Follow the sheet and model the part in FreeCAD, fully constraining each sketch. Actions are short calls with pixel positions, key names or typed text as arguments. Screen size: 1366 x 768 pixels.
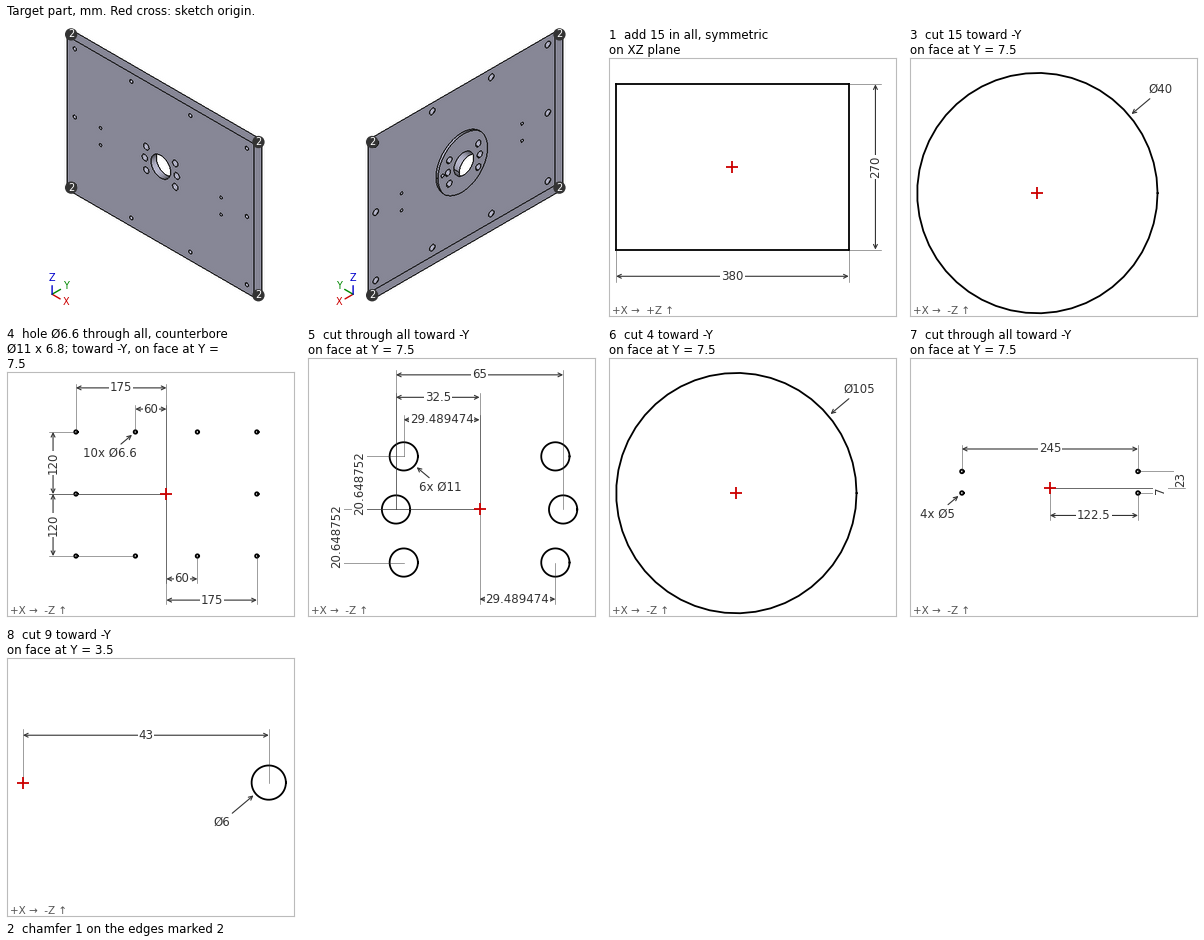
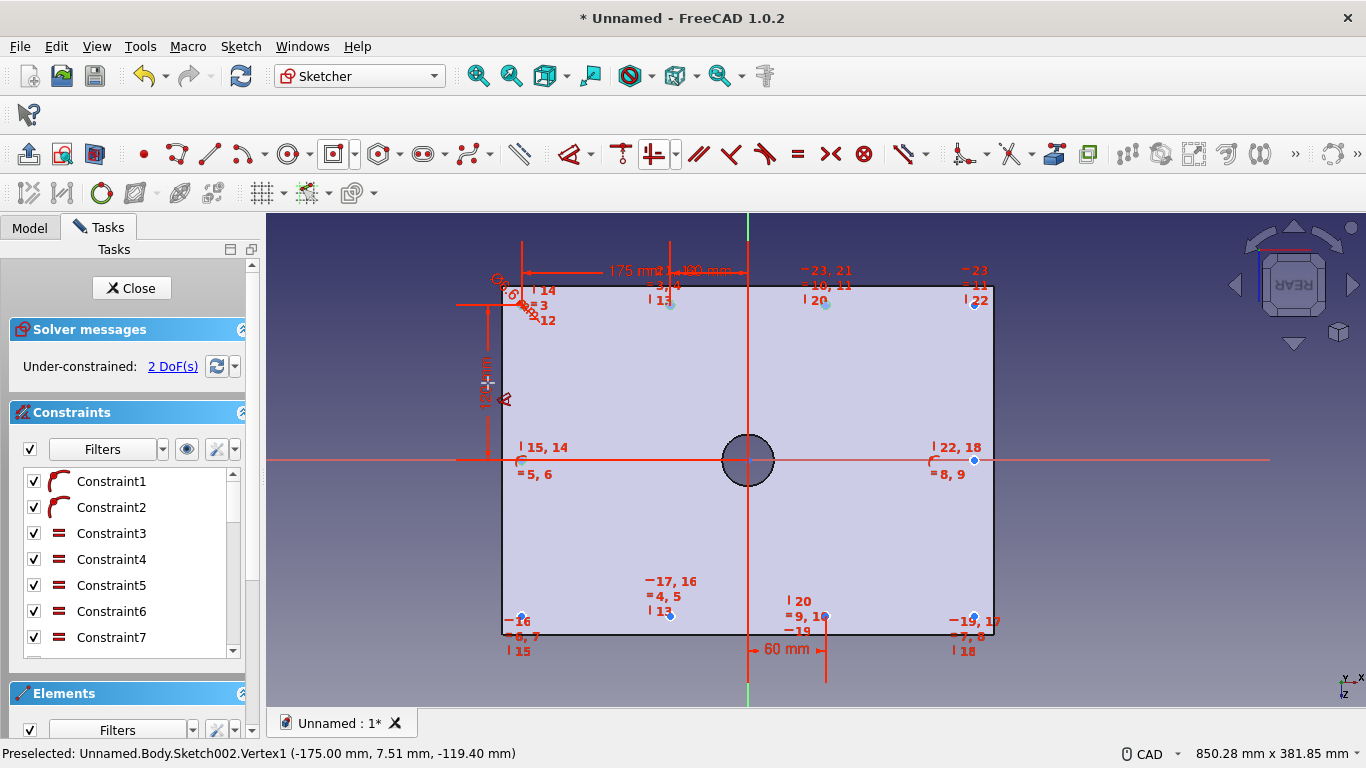
click(670, 616)
click(636, 538)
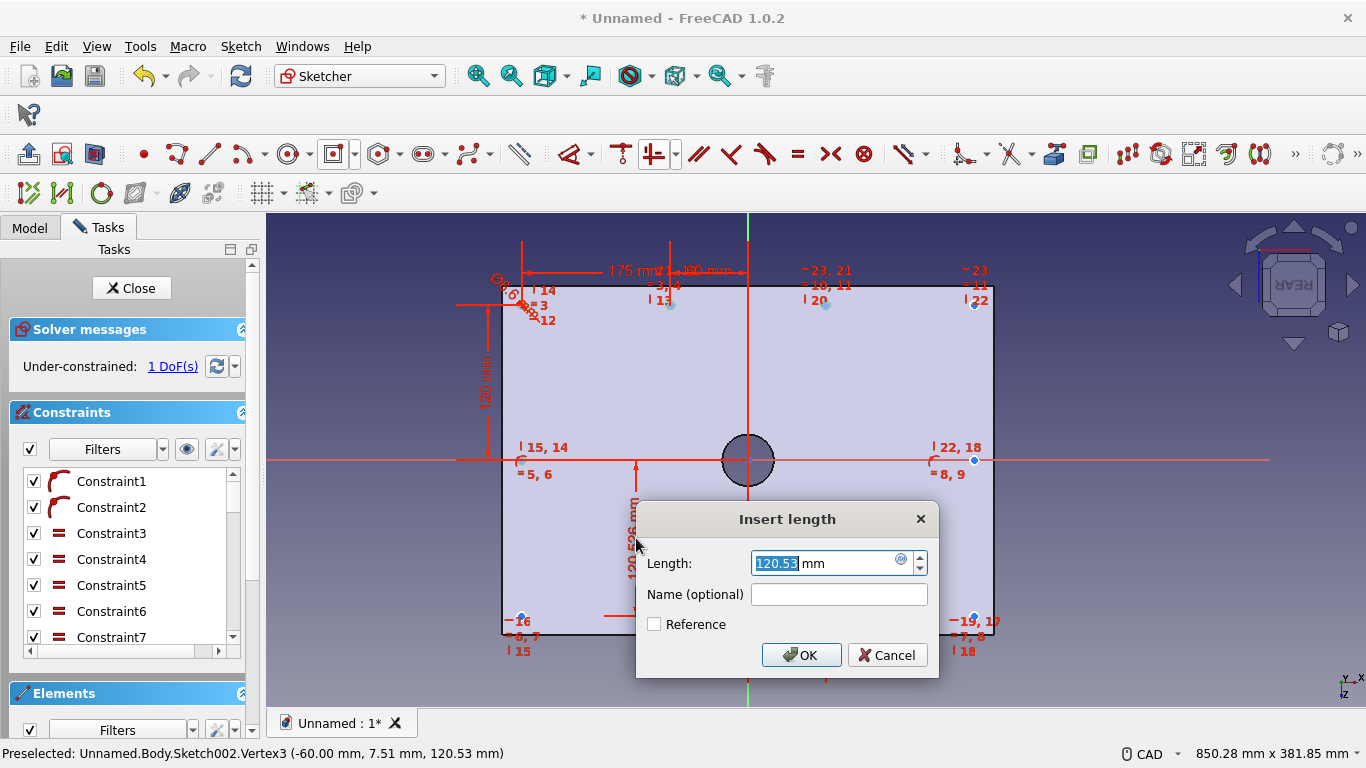
text(120)
key(Return)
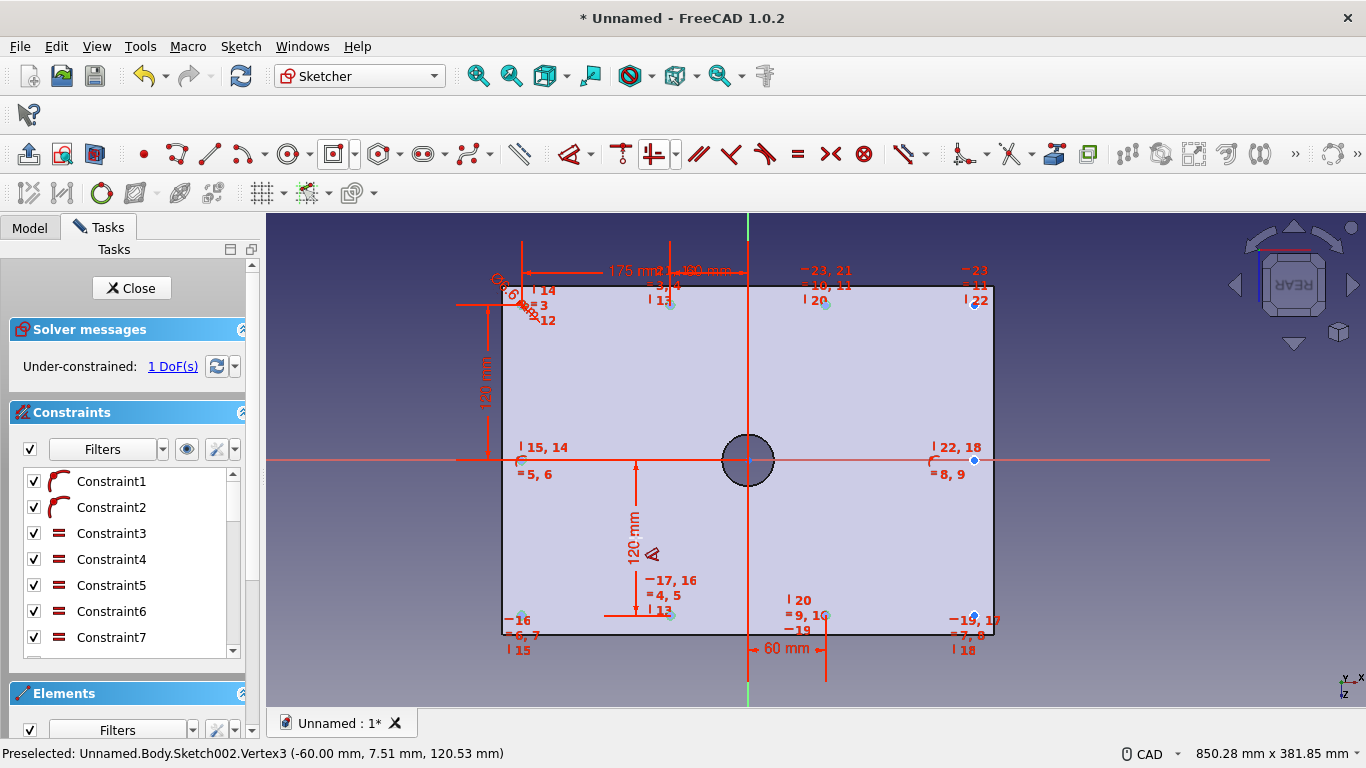
click(974, 616)
click(861, 650)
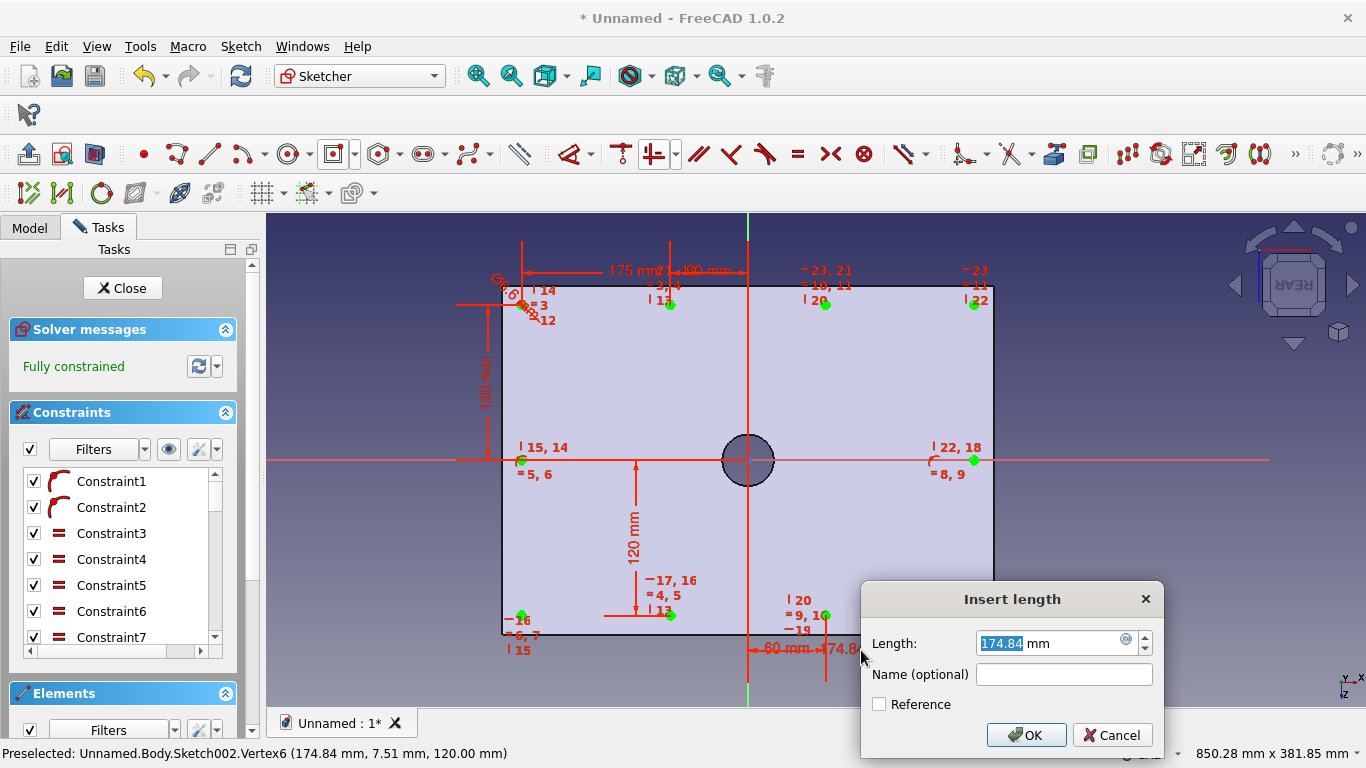
text(175)
key(Return)
key(Escape)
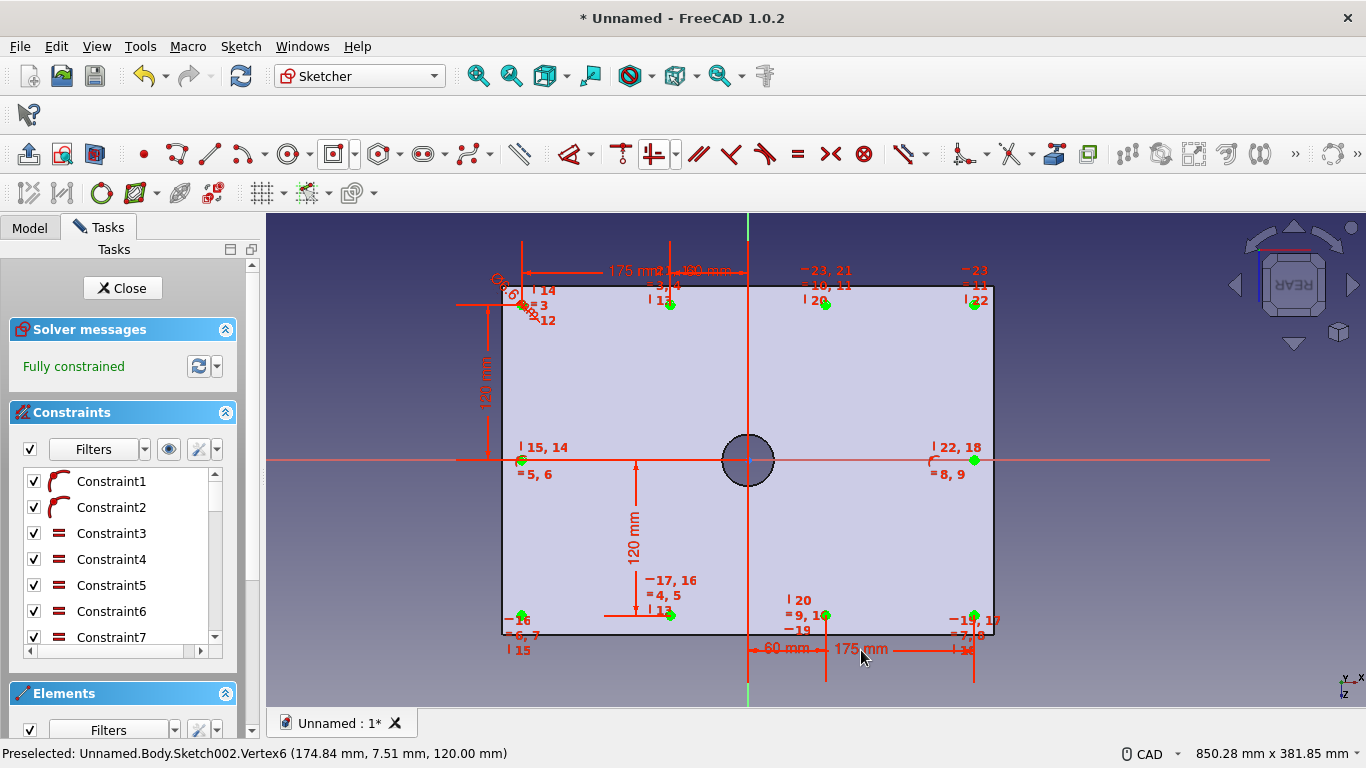
click(123, 288)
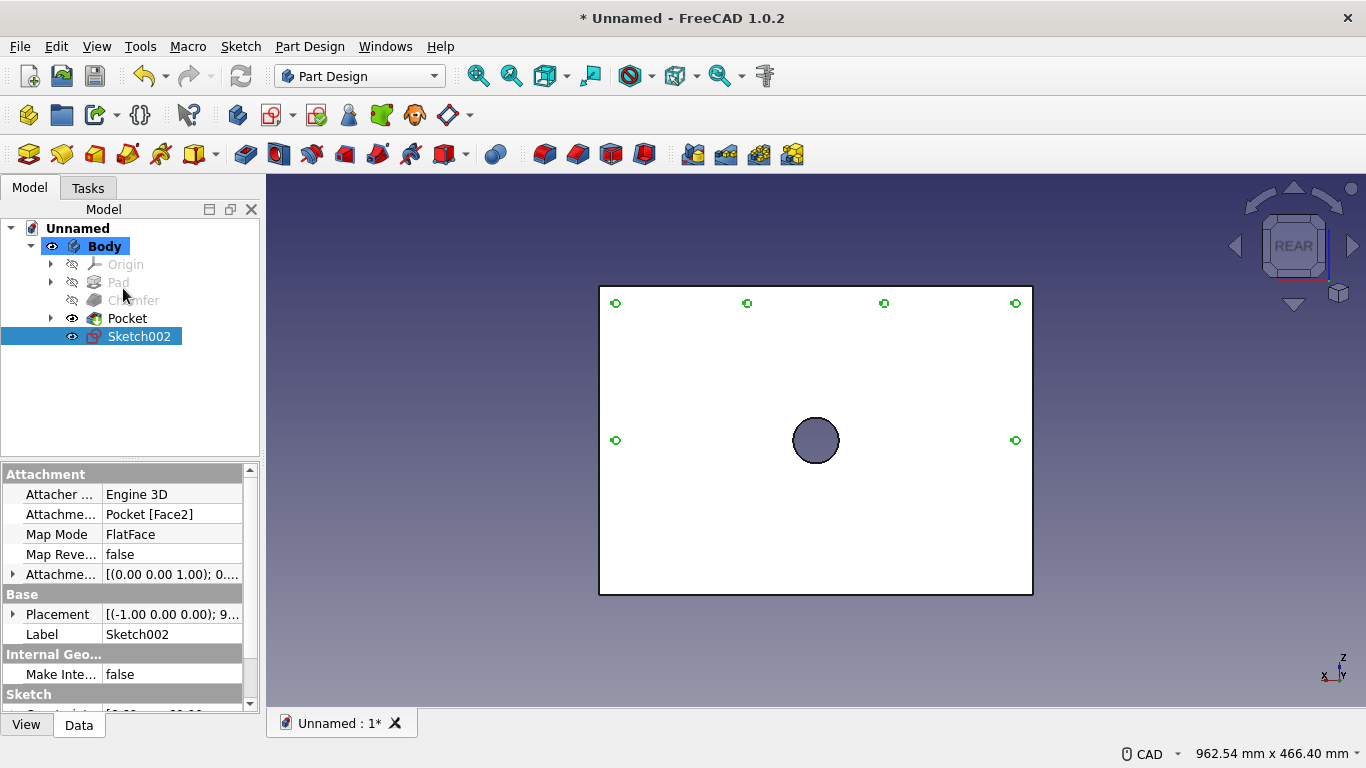
click(279, 154)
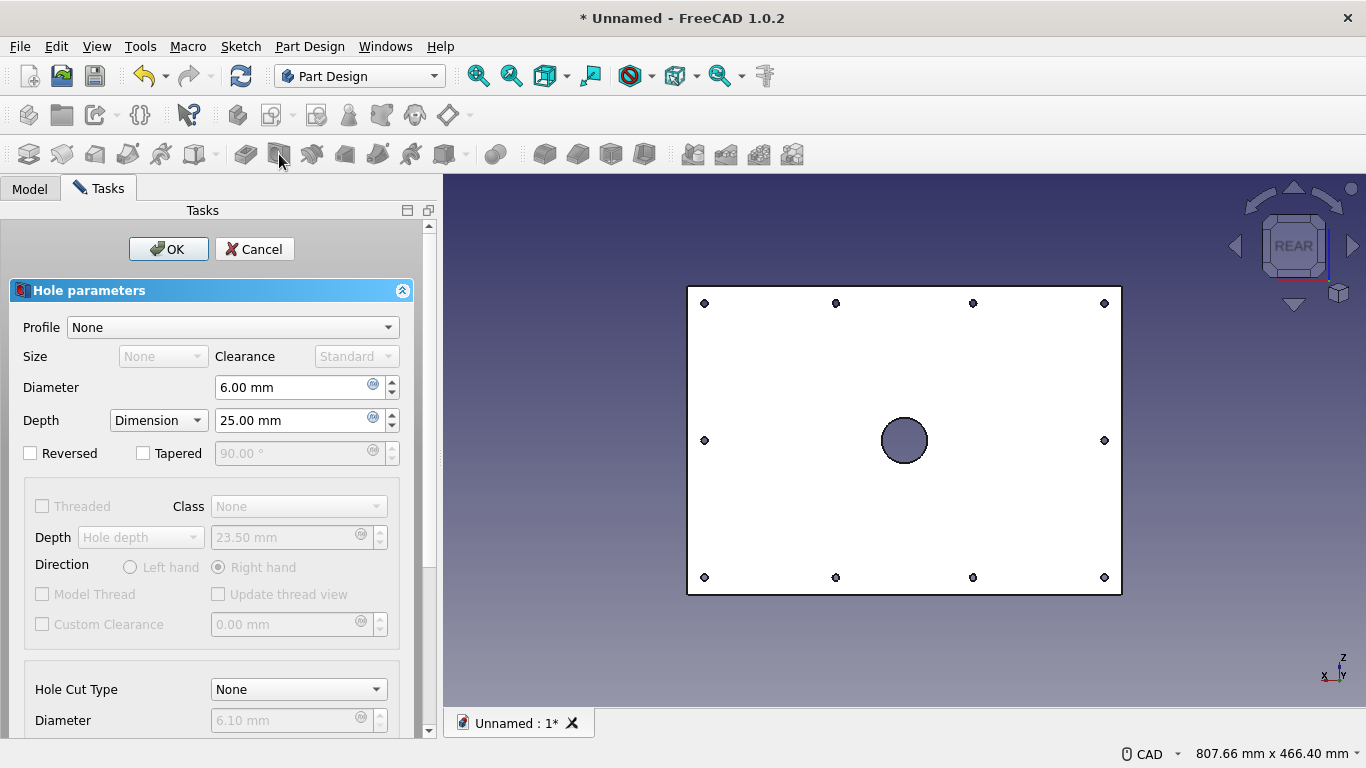
triple_click(300, 388)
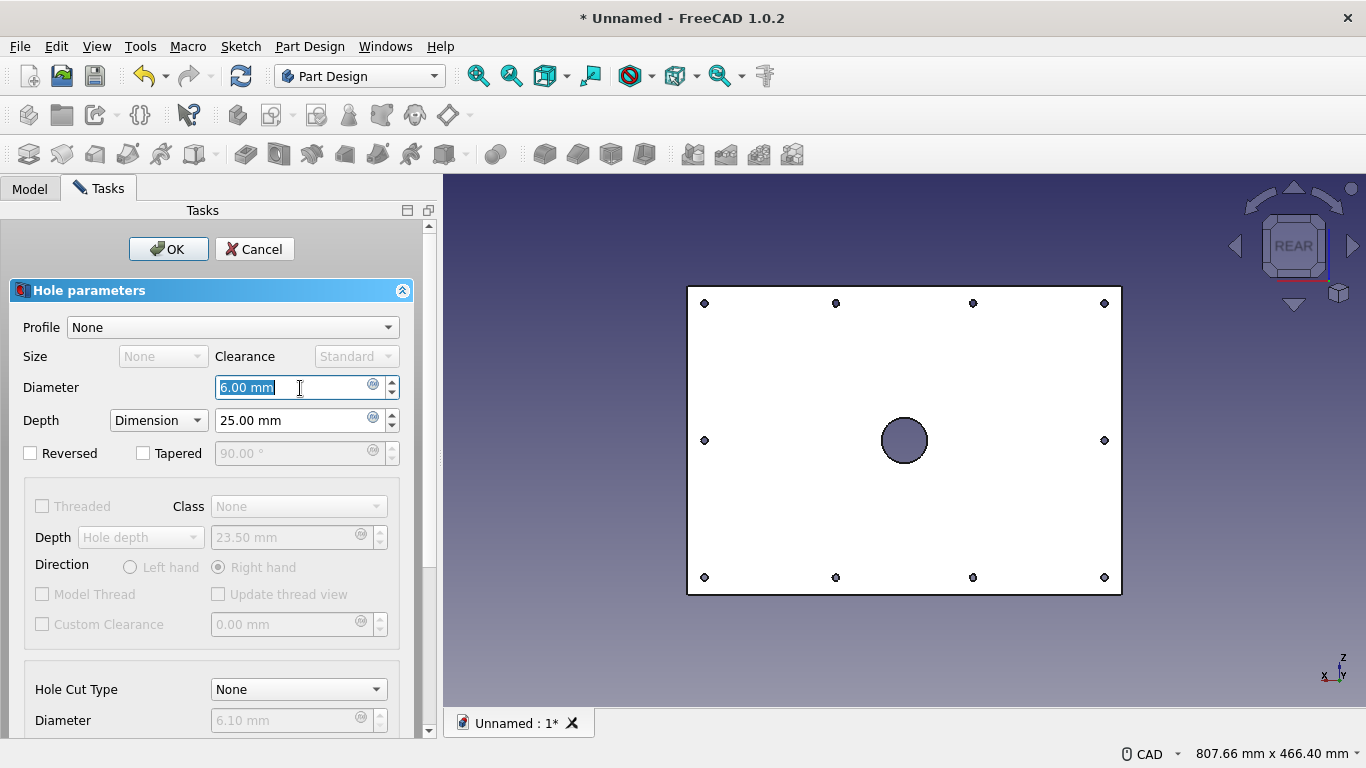
text(6.6)
key(Tab)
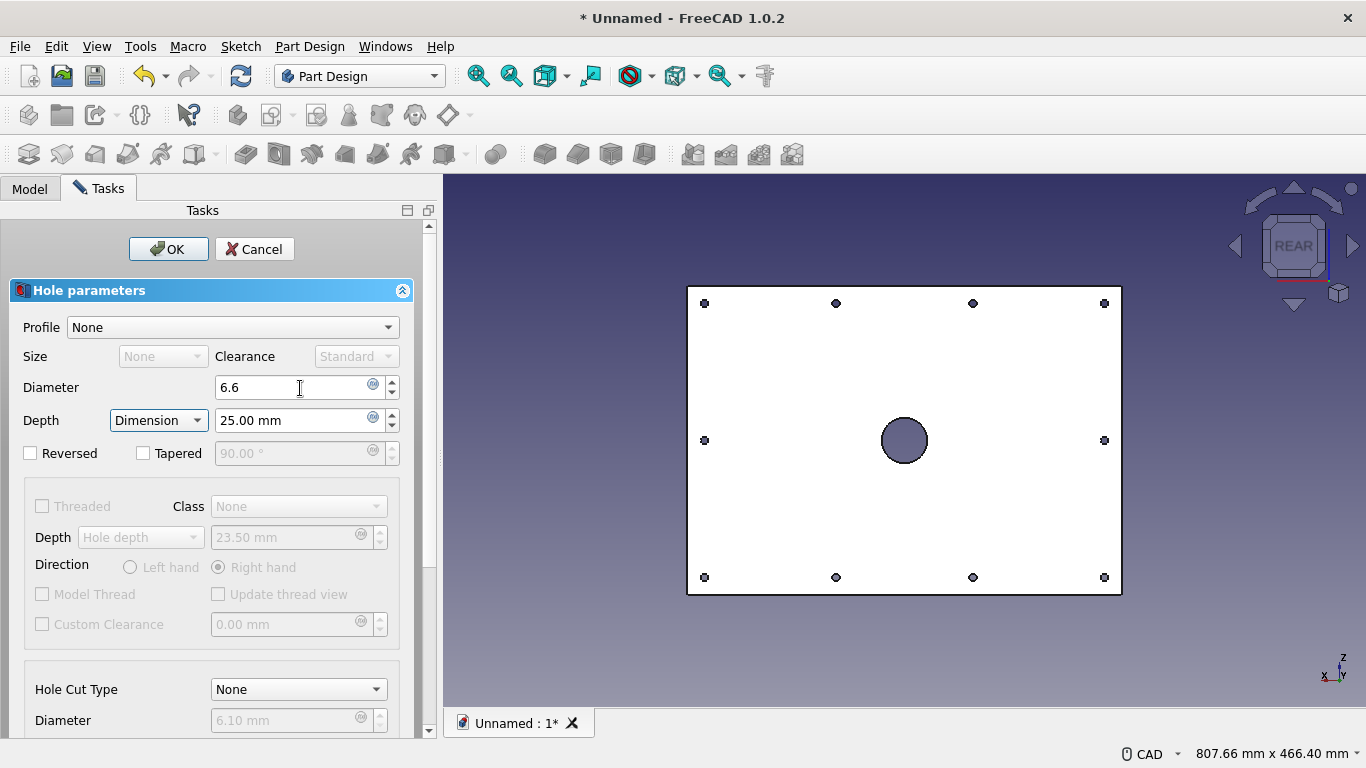
click(160, 420)